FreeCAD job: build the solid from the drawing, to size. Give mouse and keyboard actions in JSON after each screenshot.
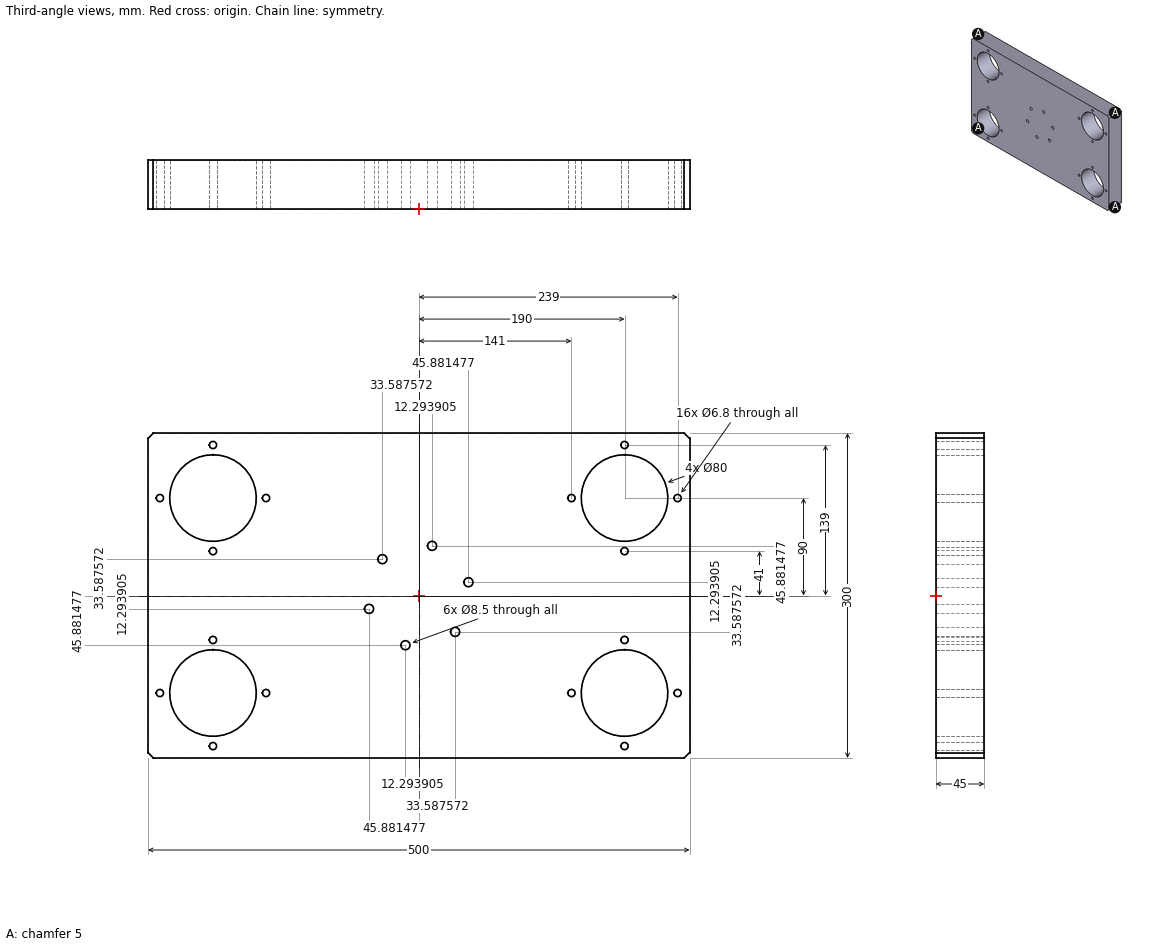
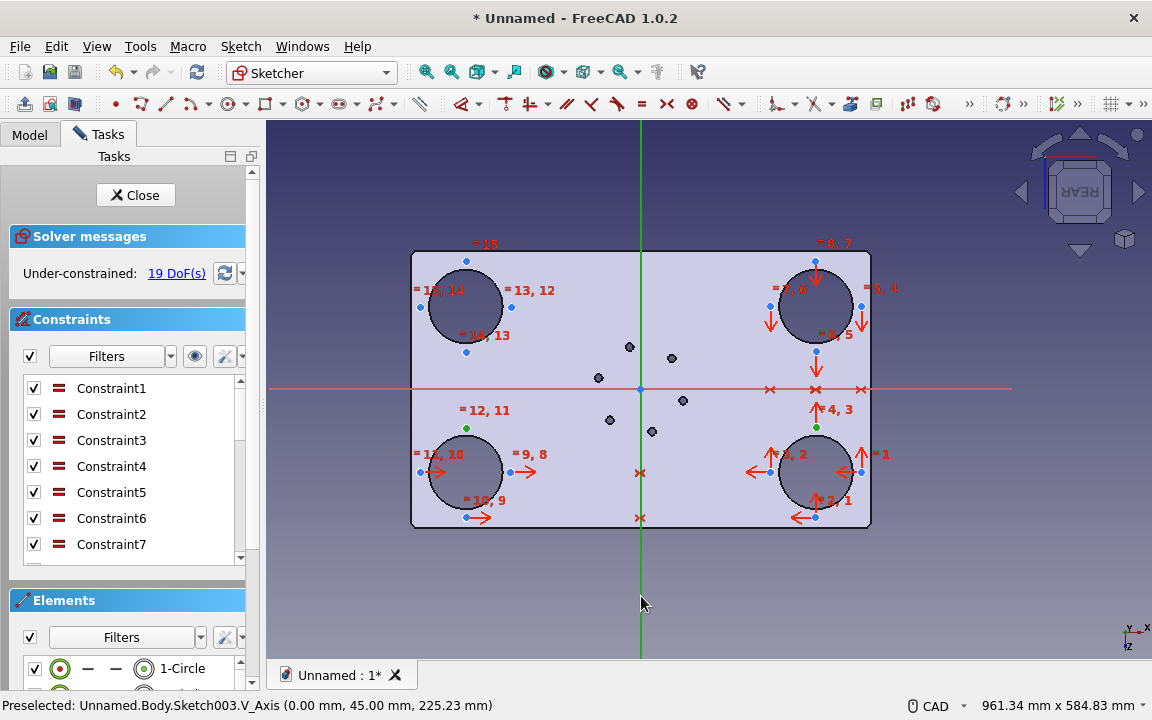
{"action": "left_click", "coordinate": [667, 104]}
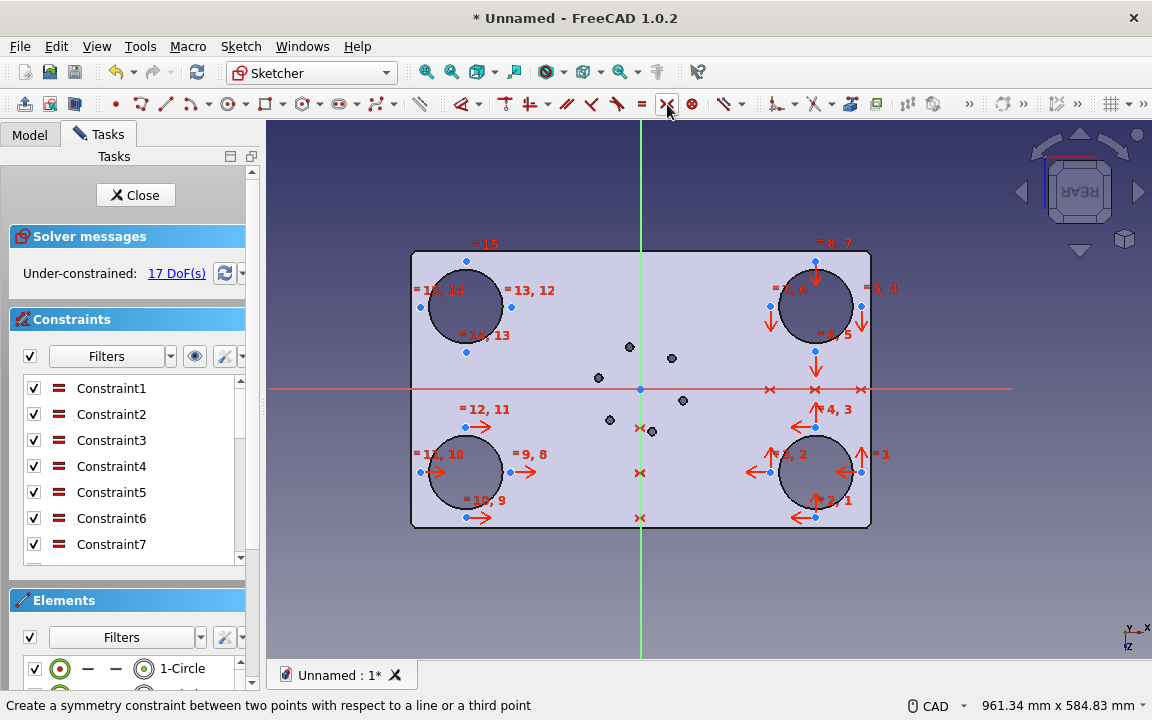
{"action": "left_click", "coordinate": [771, 307]}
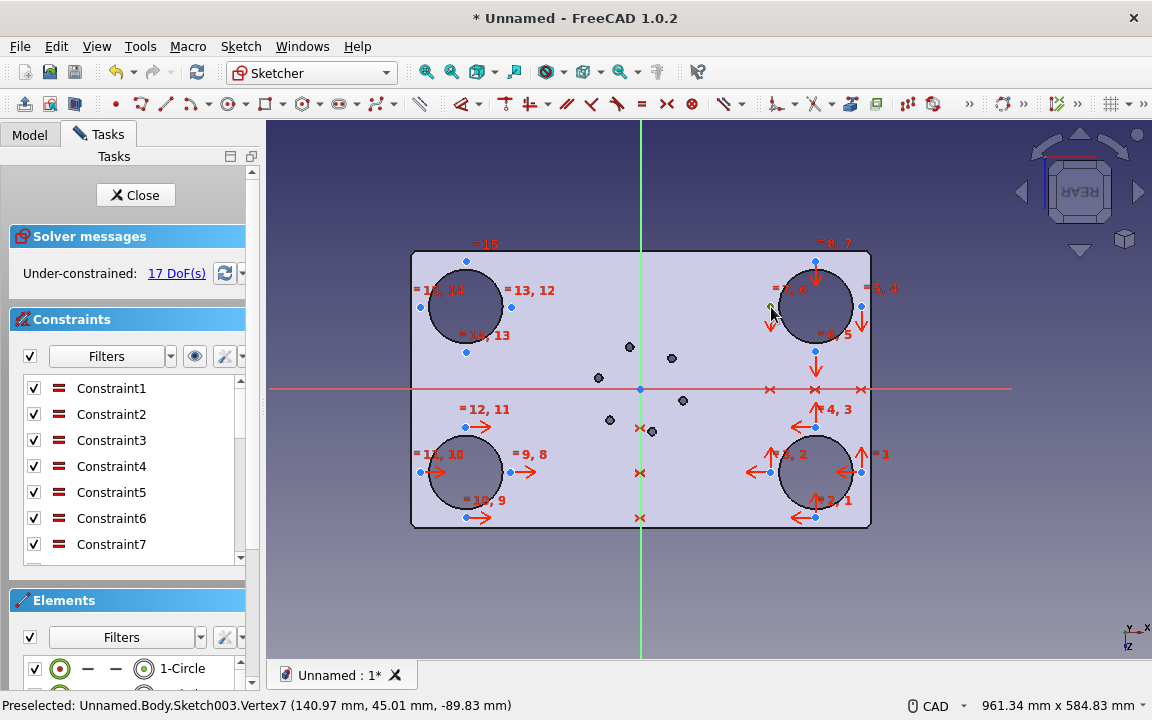
{"action": "left_click", "coordinate": [511, 308]}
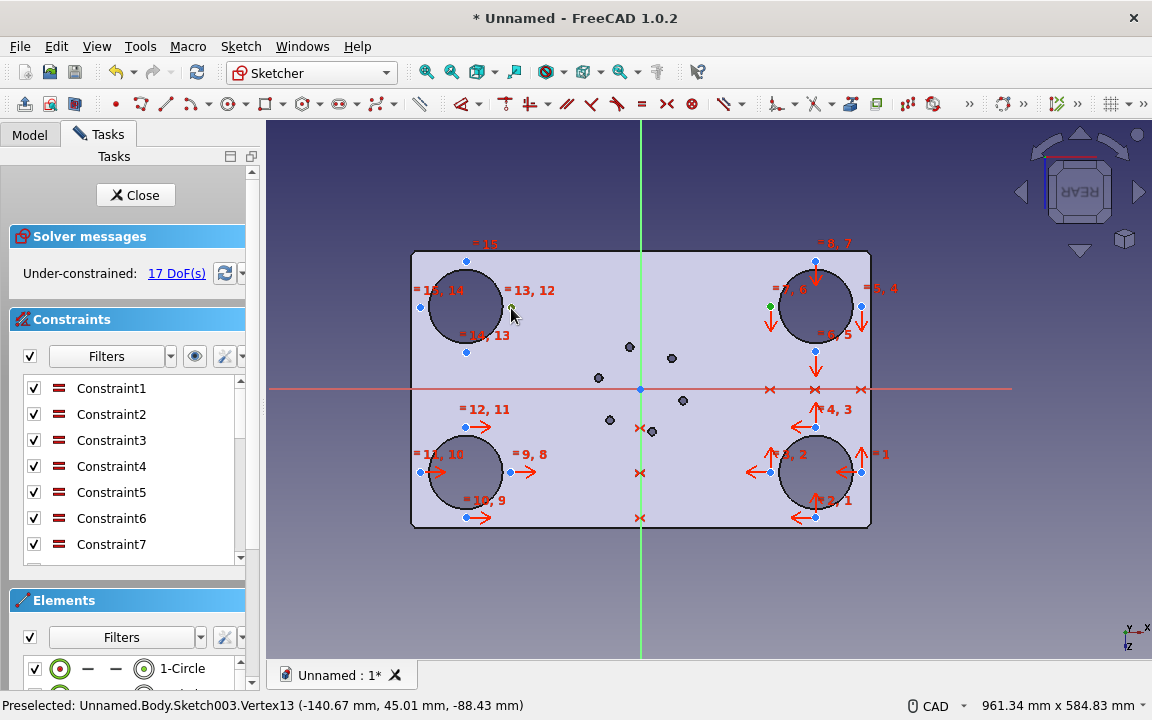
{"action": "left_click", "coordinate": [641, 596]}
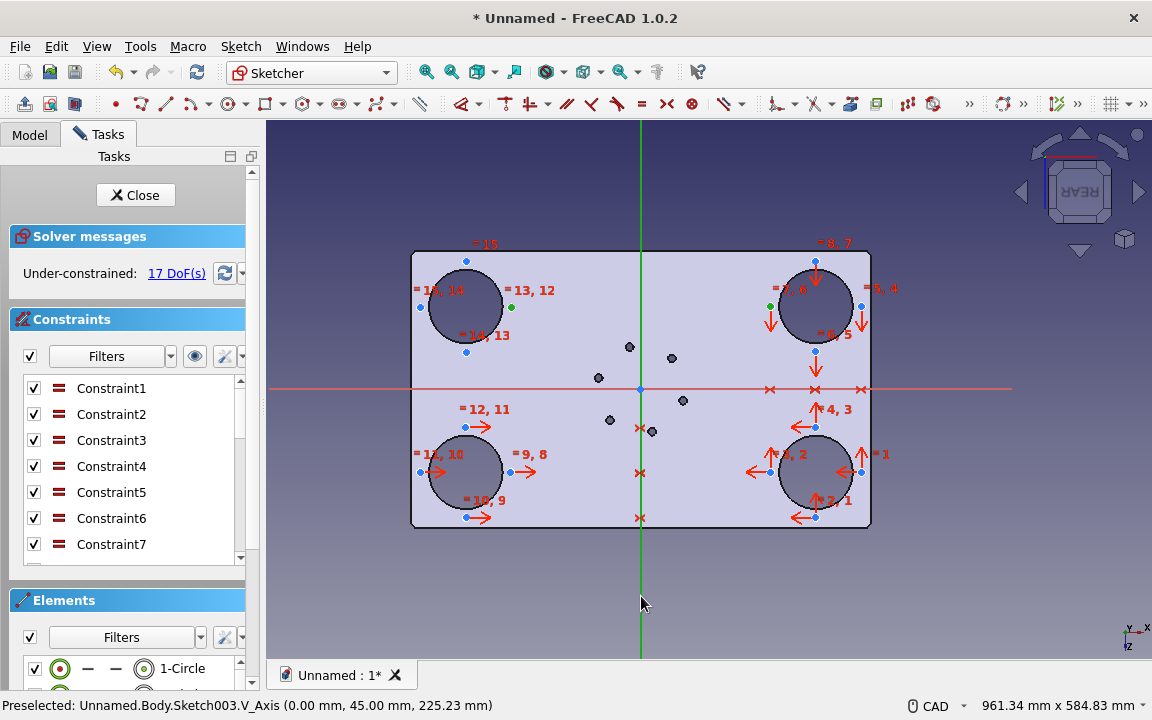
{"action": "left_click", "coordinate": [667, 104]}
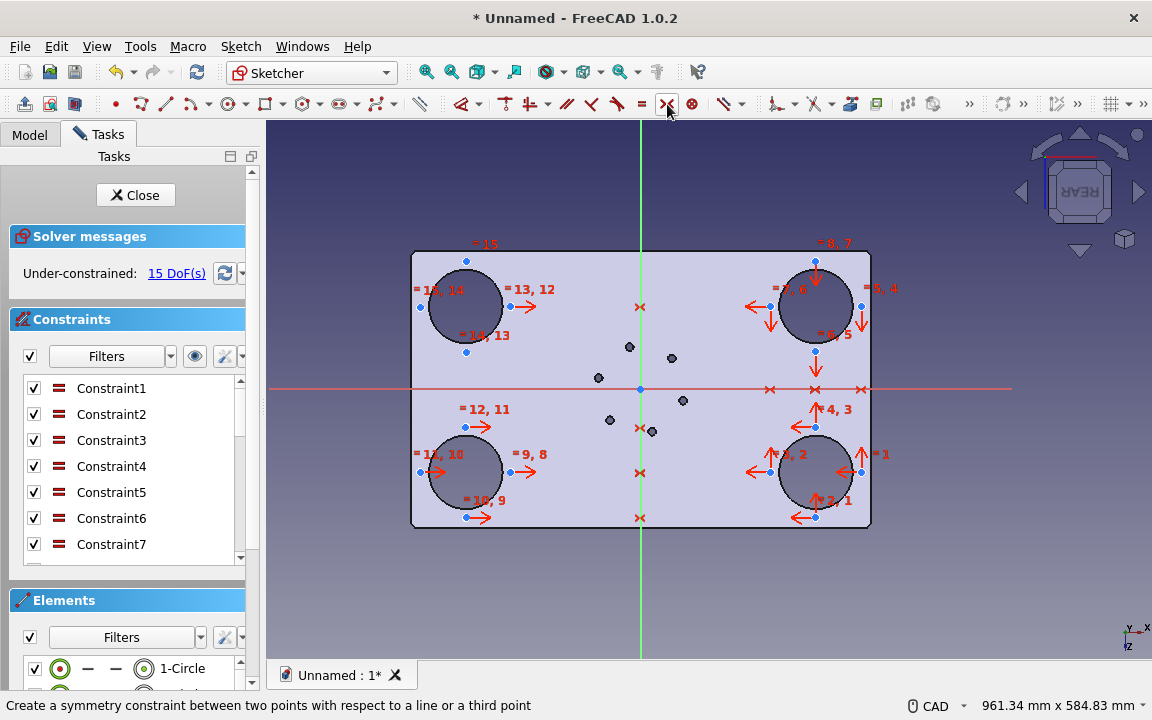
{"action": "left_click", "coordinate": [816, 352]}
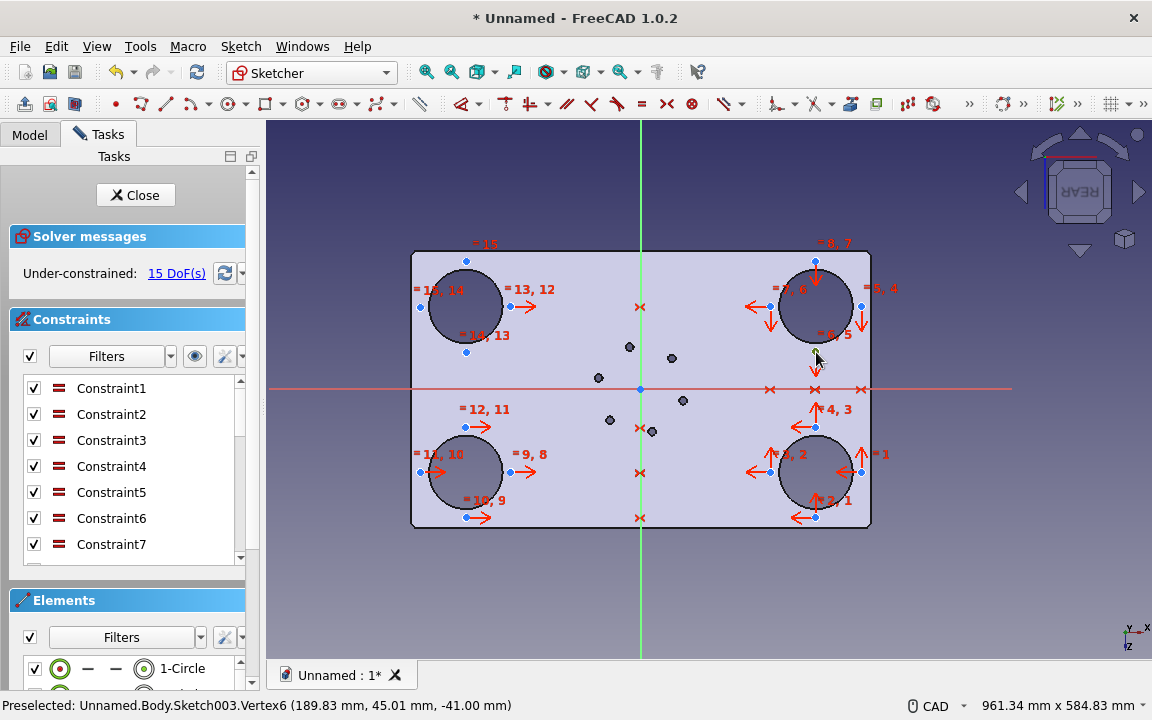
{"action": "left_click", "coordinate": [466, 353]}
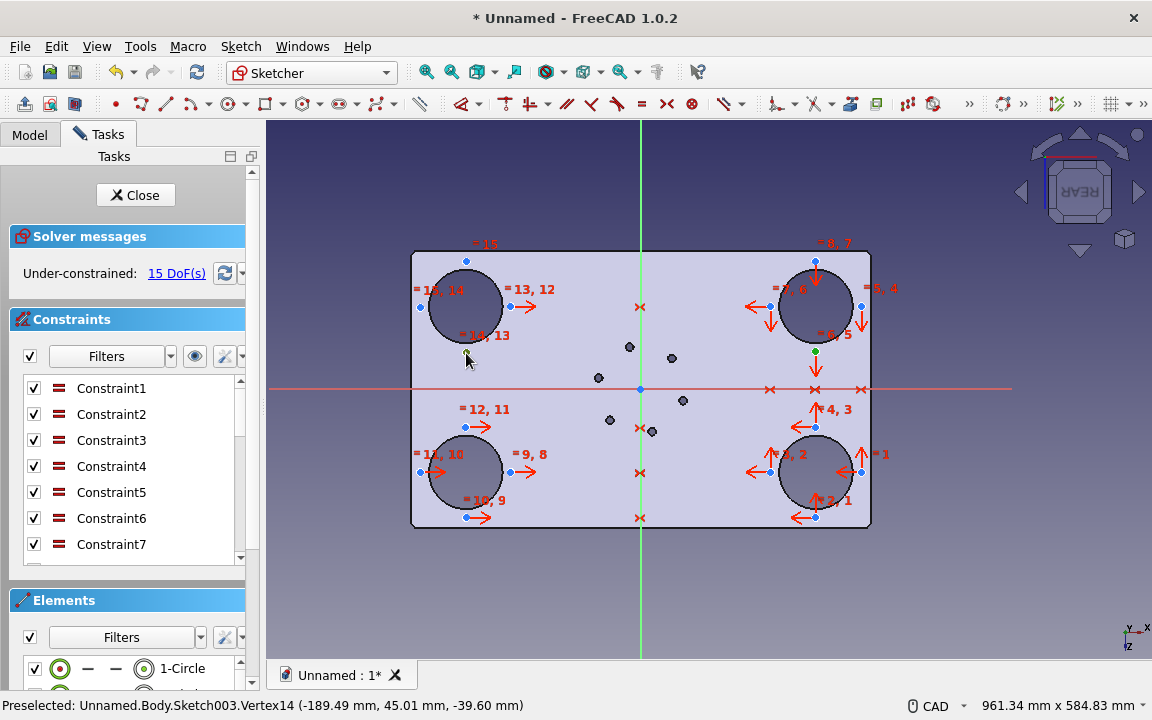
{"action": "left_click", "coordinate": [641, 596]}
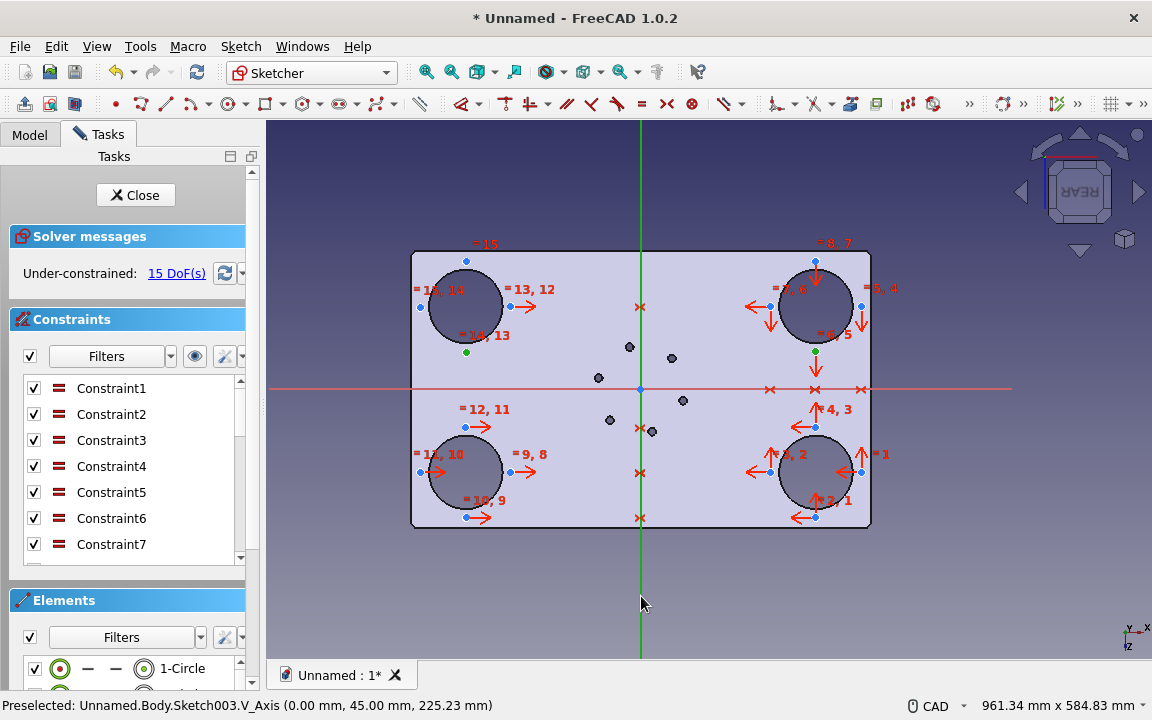
{"action": "left_click", "coordinate": [667, 104]}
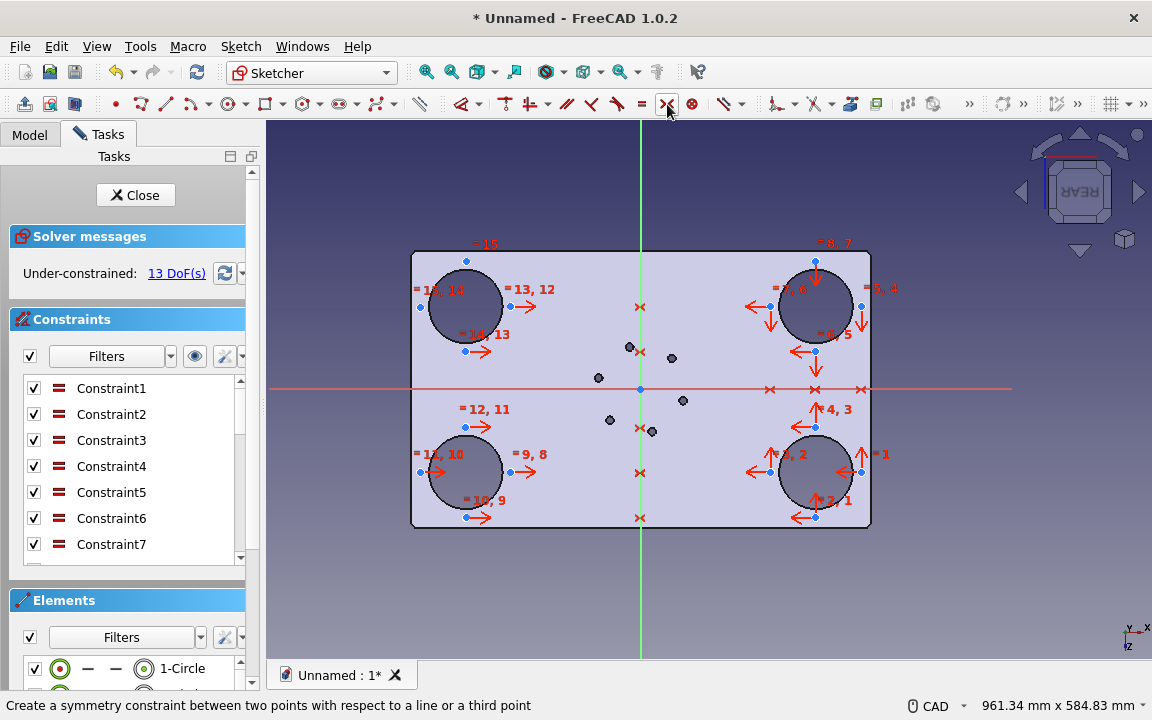
{"action": "left_click", "coordinate": [862, 307]}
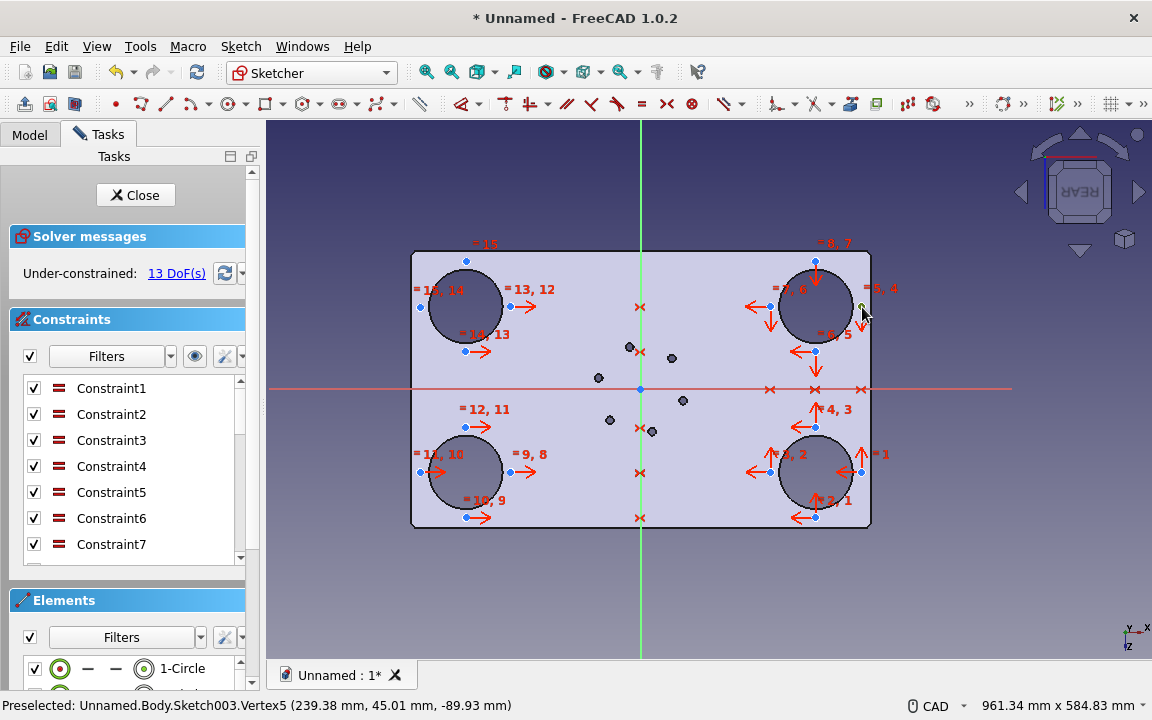
{"action": "left_click", "coordinate": [420, 308]}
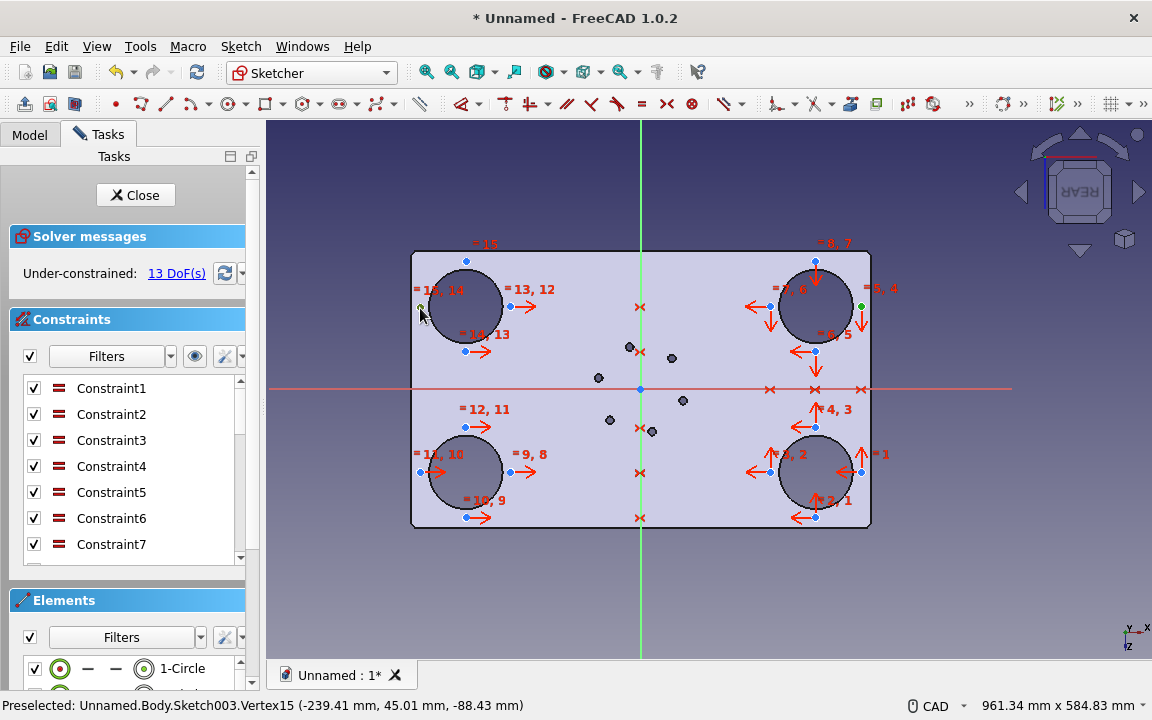
{"action": "left_click", "coordinate": [641, 596]}